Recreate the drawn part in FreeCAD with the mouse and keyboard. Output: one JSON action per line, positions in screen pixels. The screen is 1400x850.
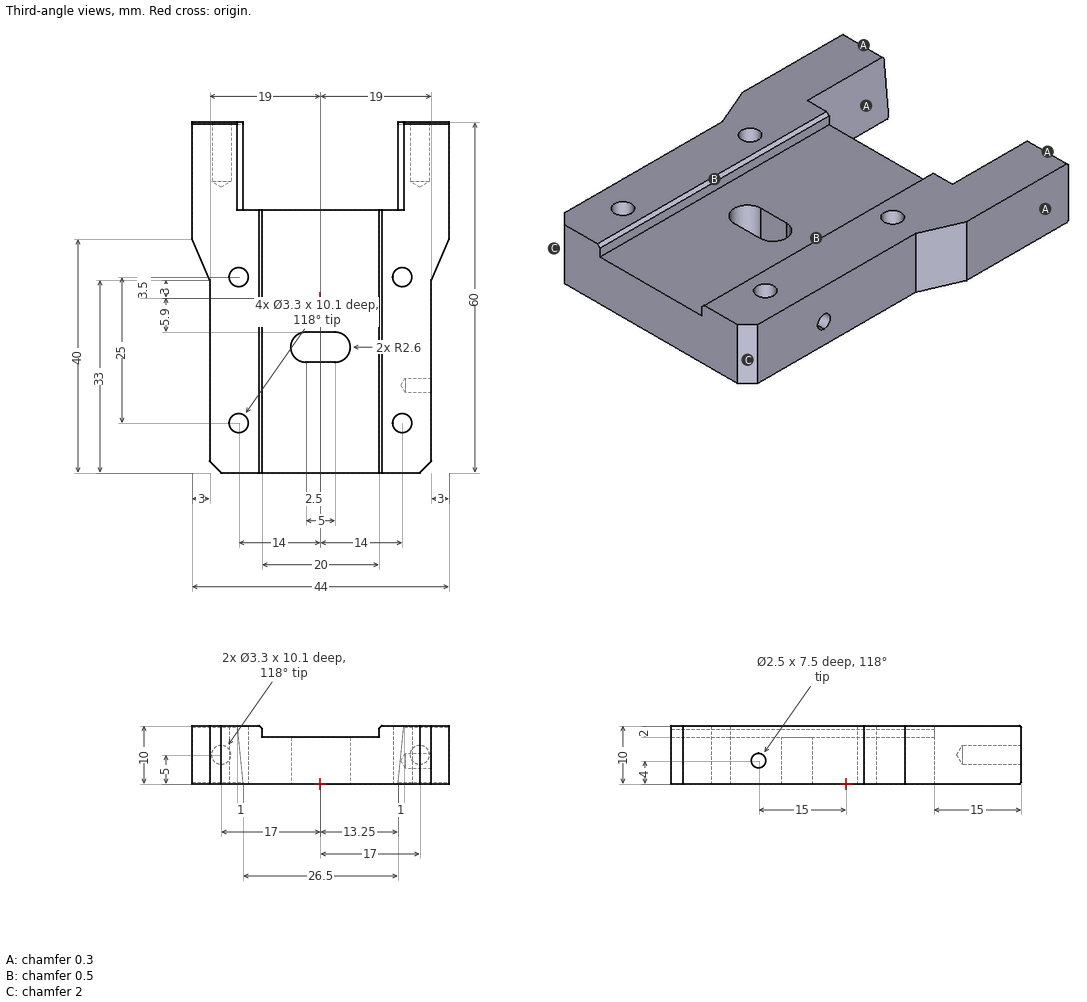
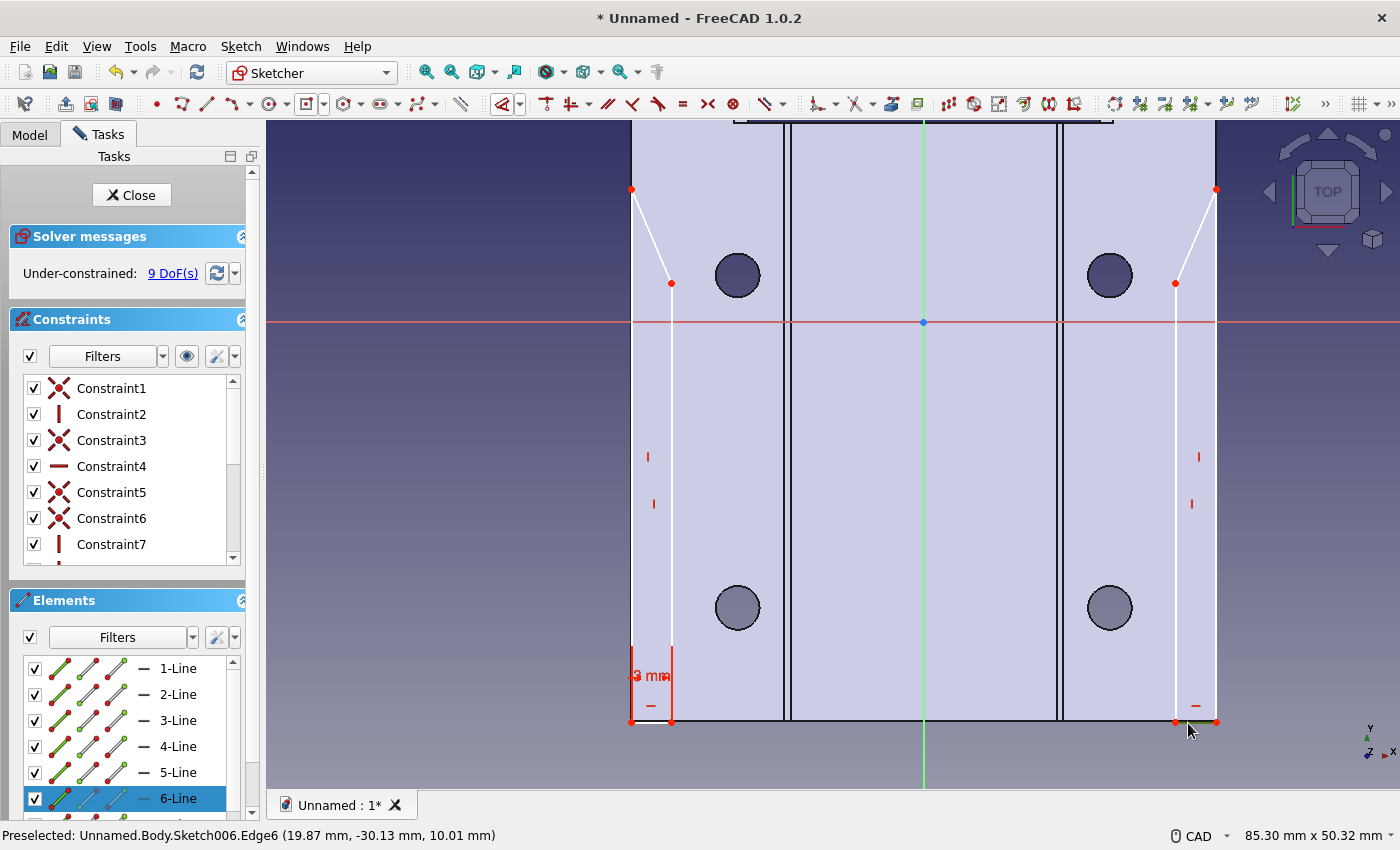
{"action": "key", "text": "l"}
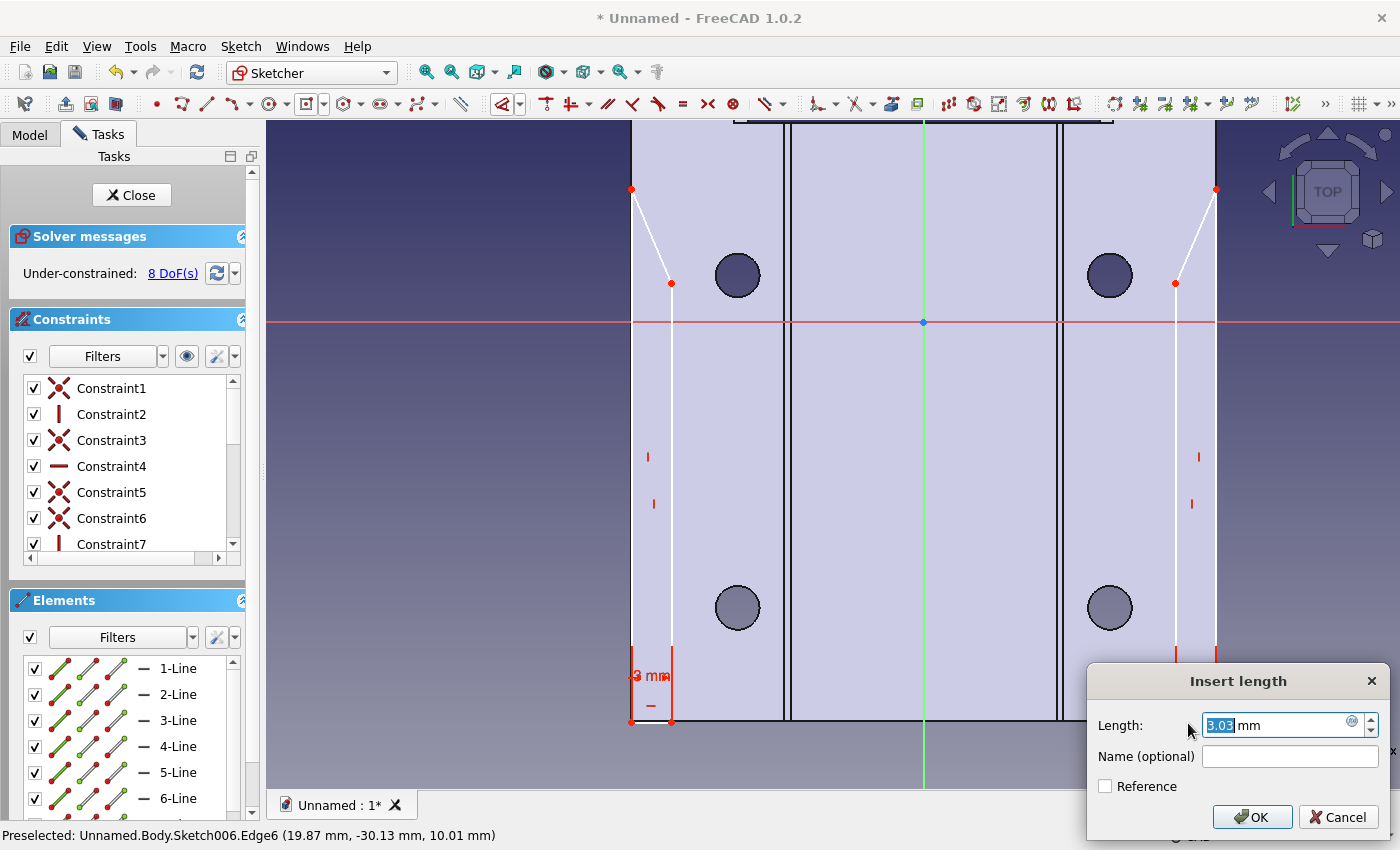
{"action": "type", "text": "3"}
{"action": "key", "text": "Return"}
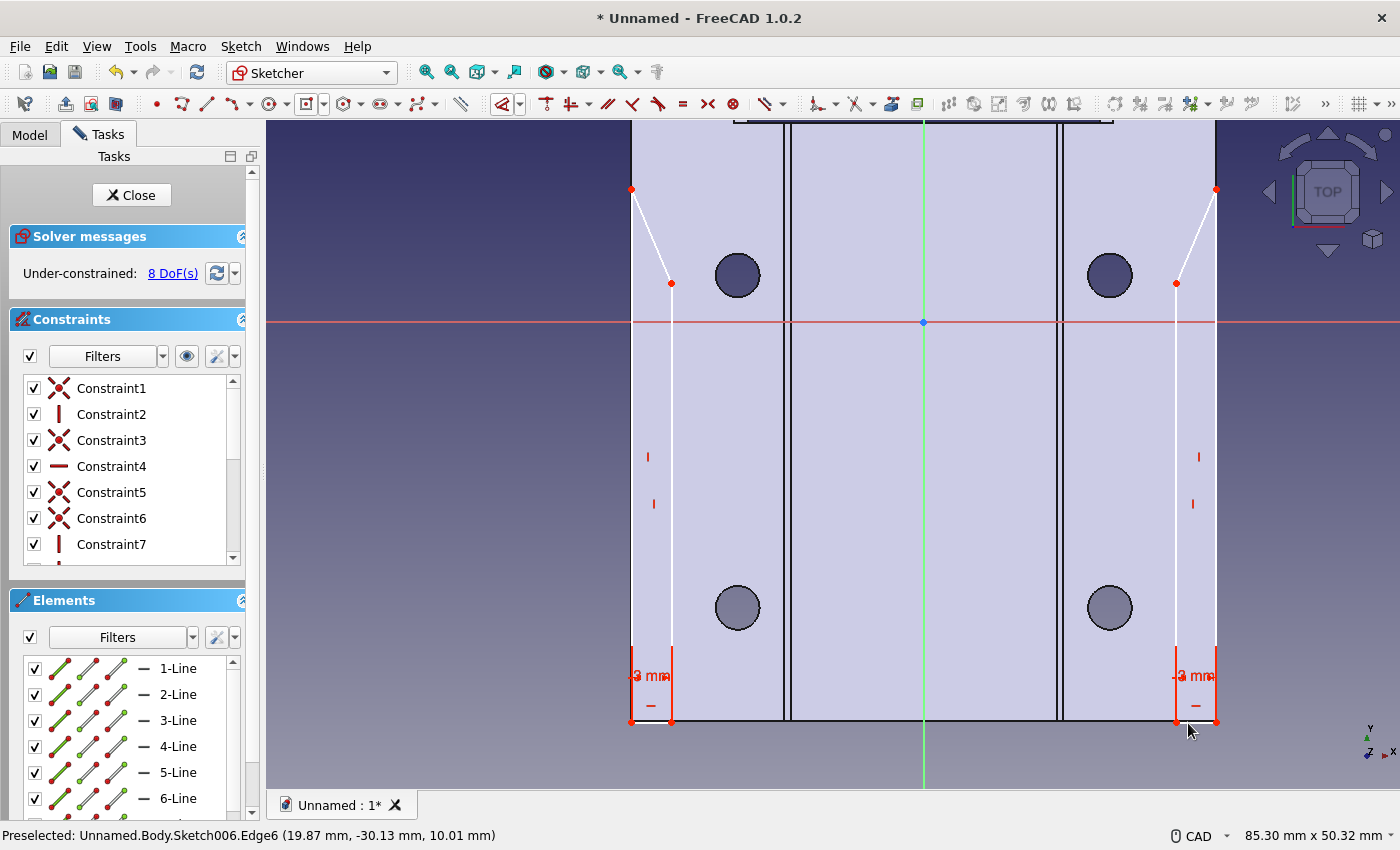
{"action": "left_click", "coordinate": [632, 350]}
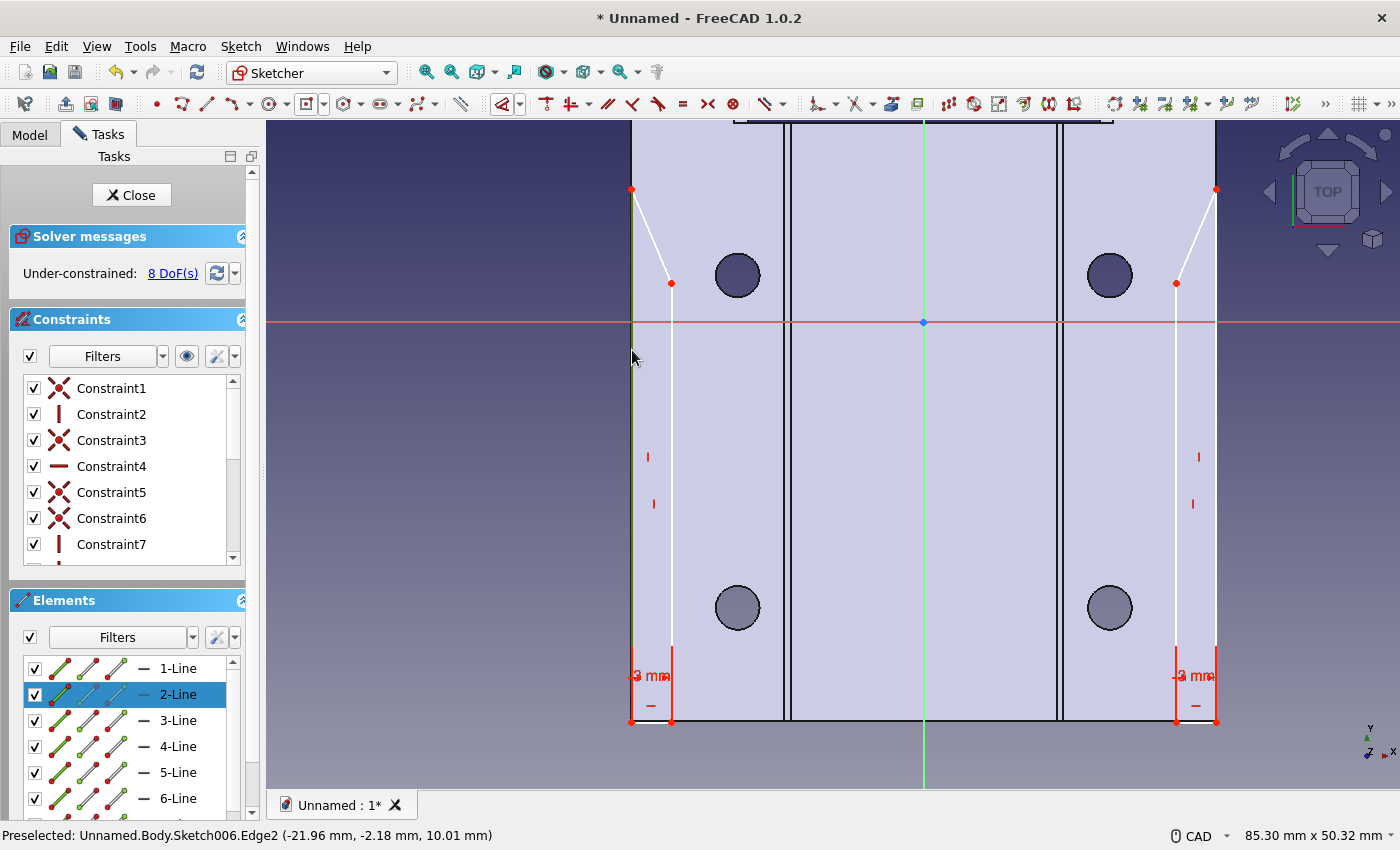
{"action": "left_click", "coordinate": [520, 104]}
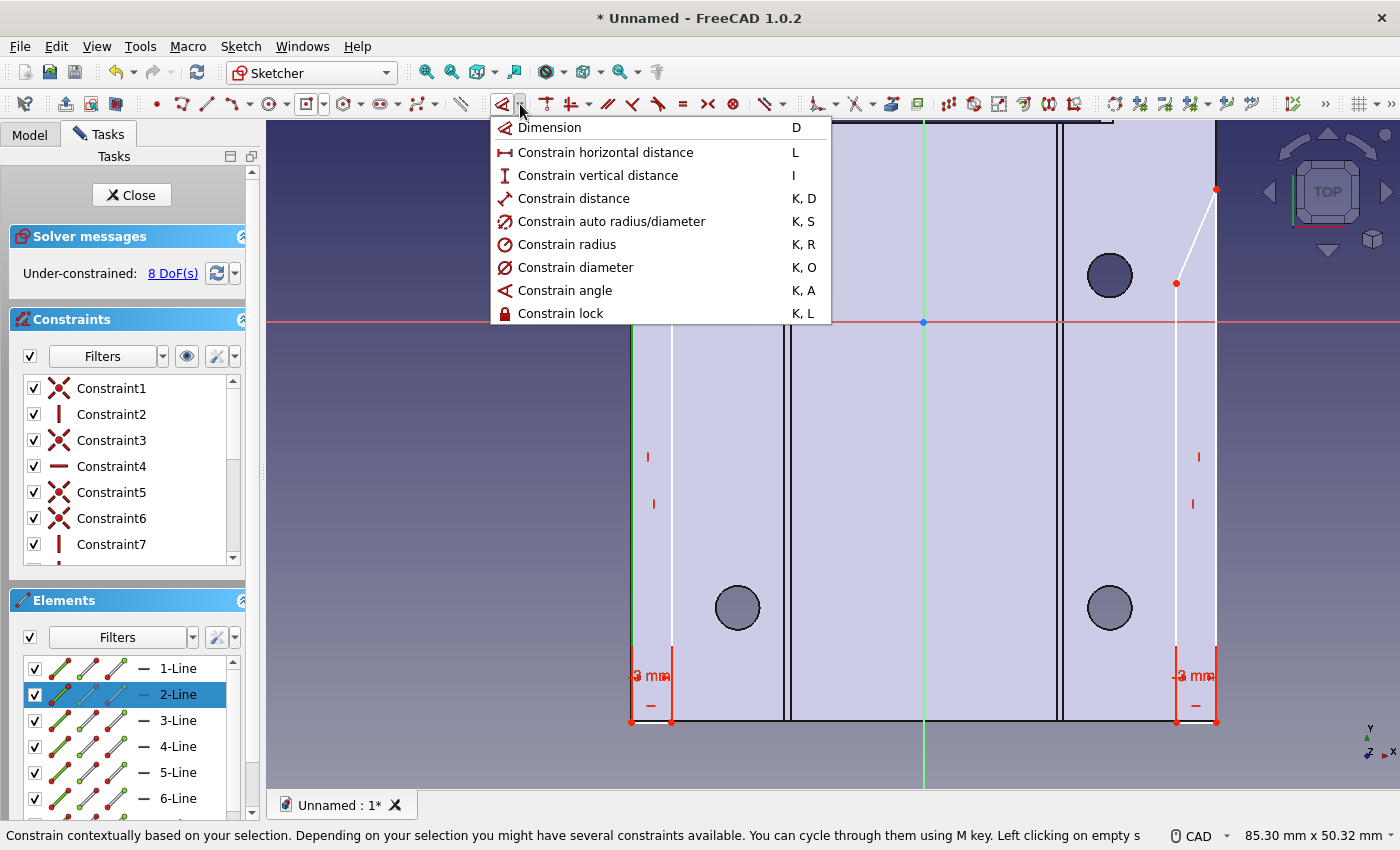
{"action": "left_click", "coordinate": [661, 176]}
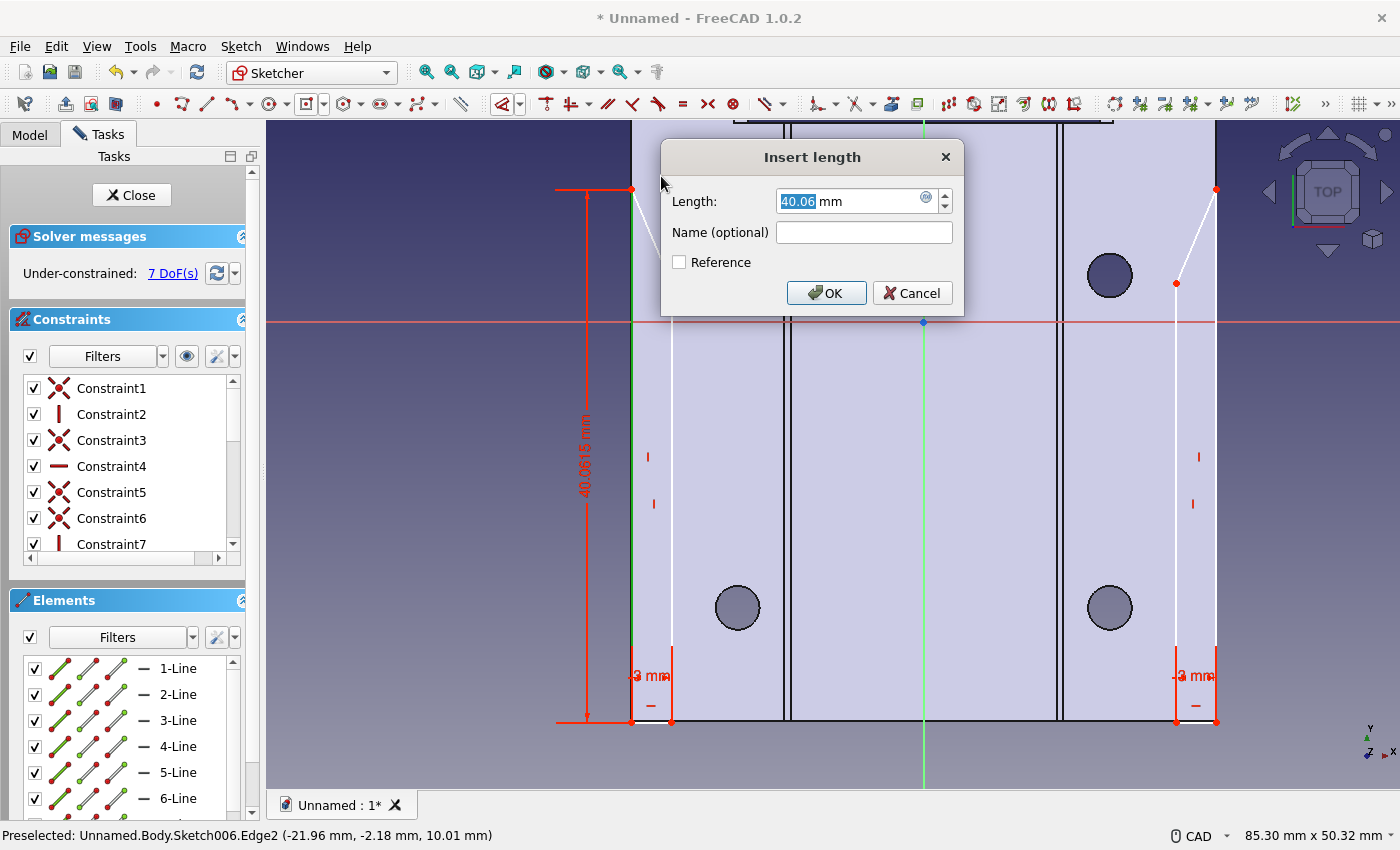
{"action": "type", "text": "40"}
{"action": "key", "text": "Return"}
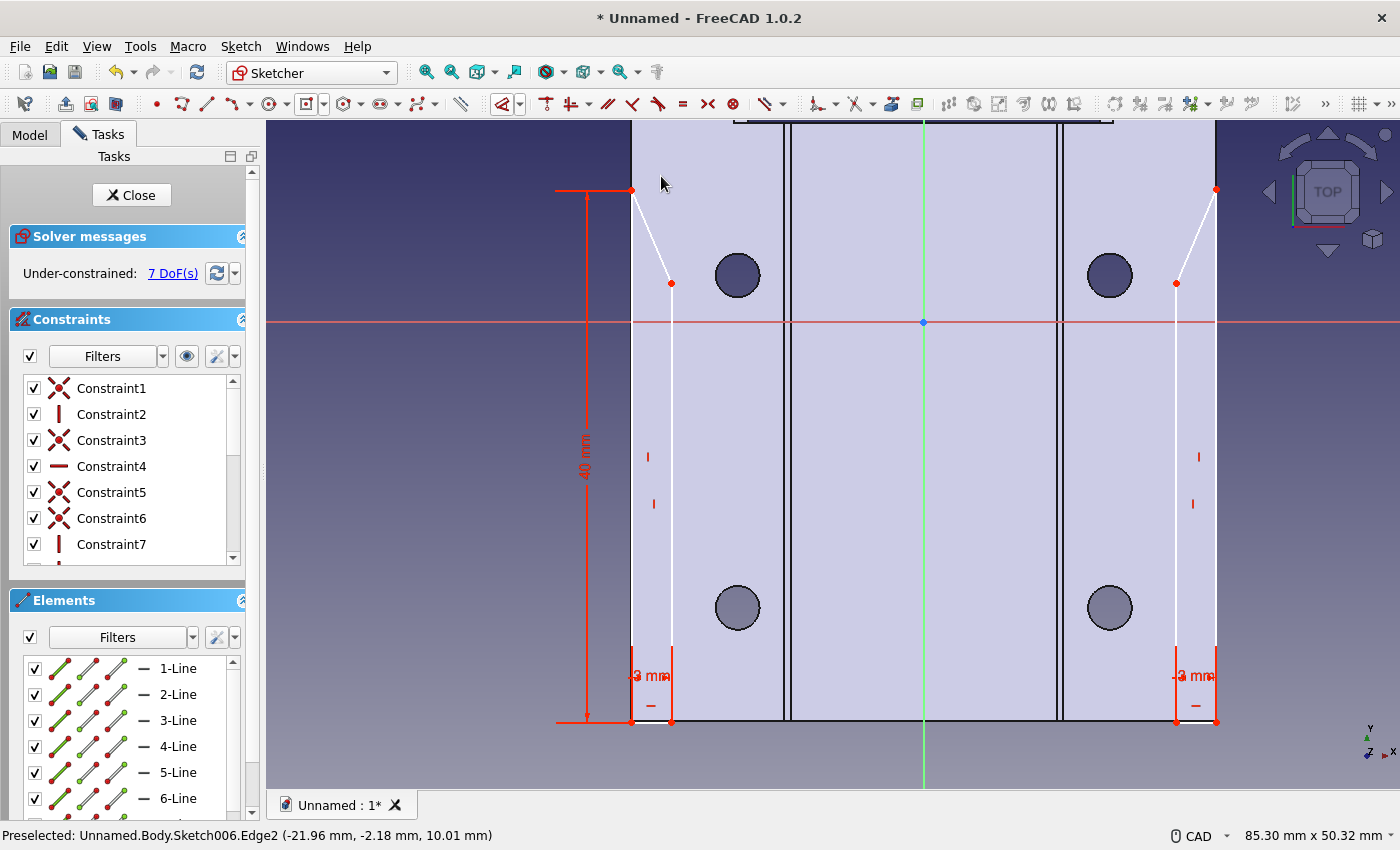
{"action": "left_click", "coordinate": [672, 591]}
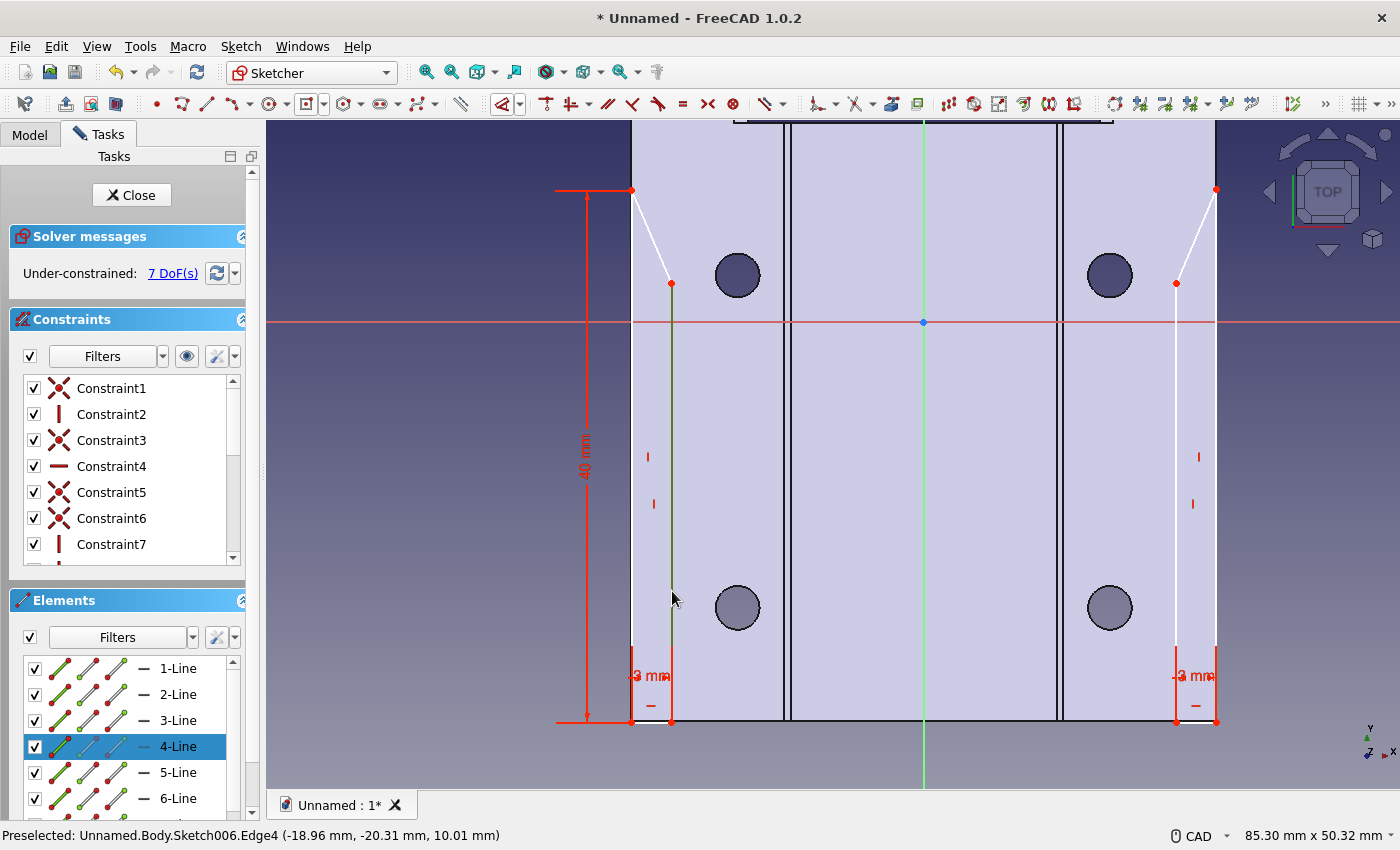
{"action": "key", "text": "i"}